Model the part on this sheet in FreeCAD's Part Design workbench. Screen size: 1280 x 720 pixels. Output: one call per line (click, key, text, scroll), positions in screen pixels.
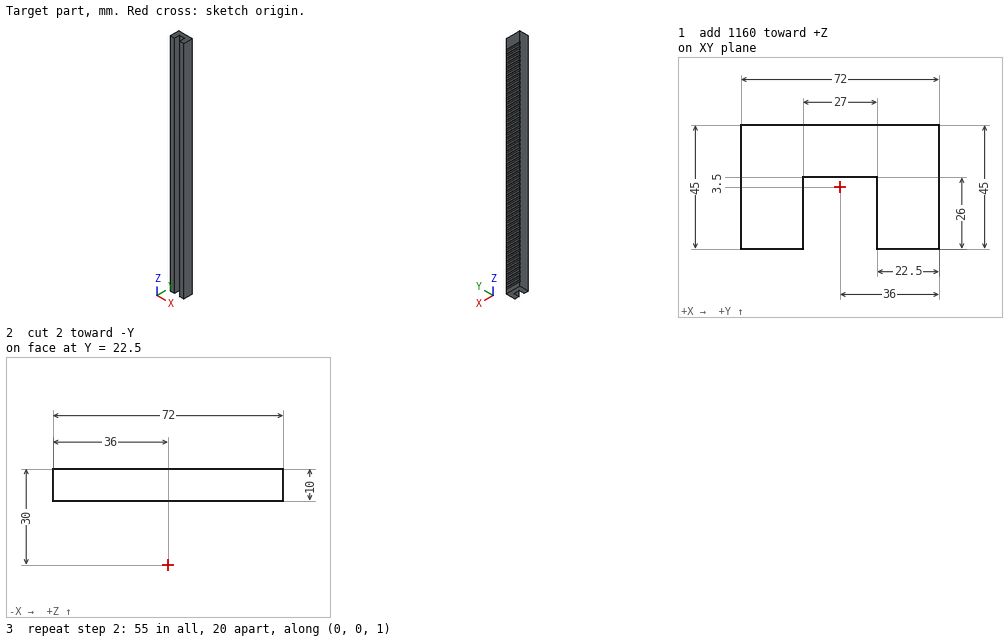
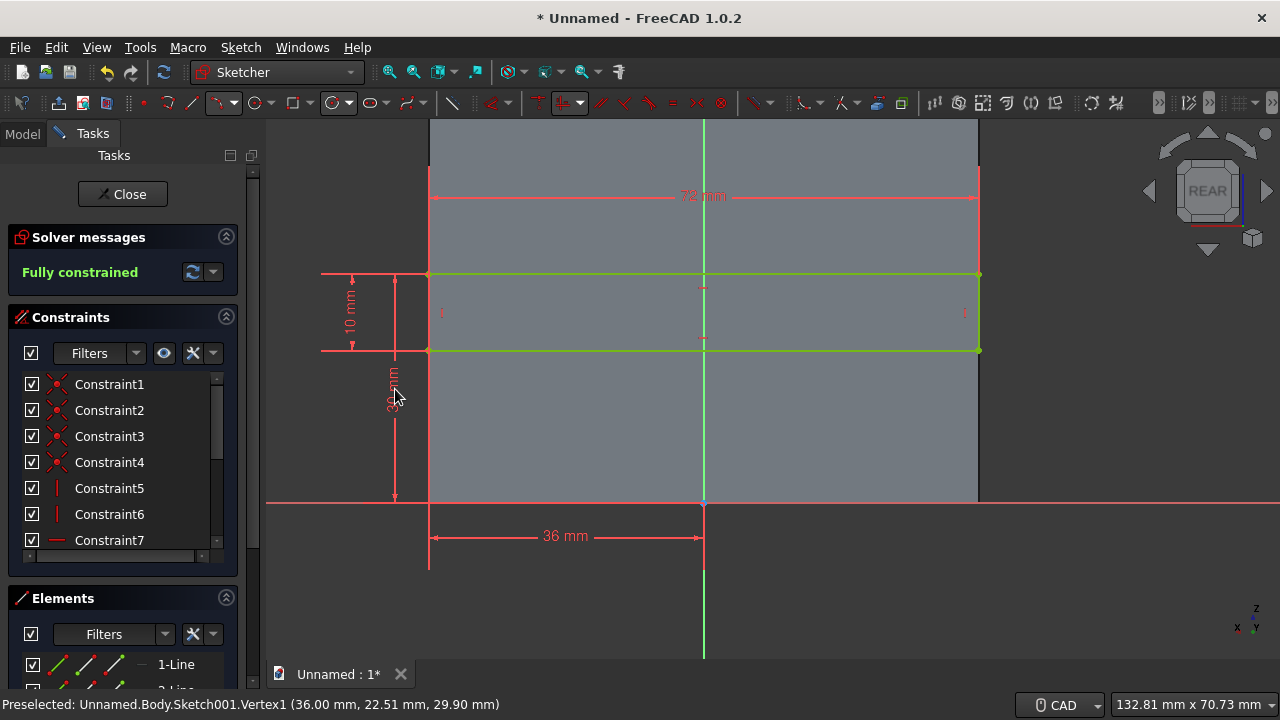
click(123, 194)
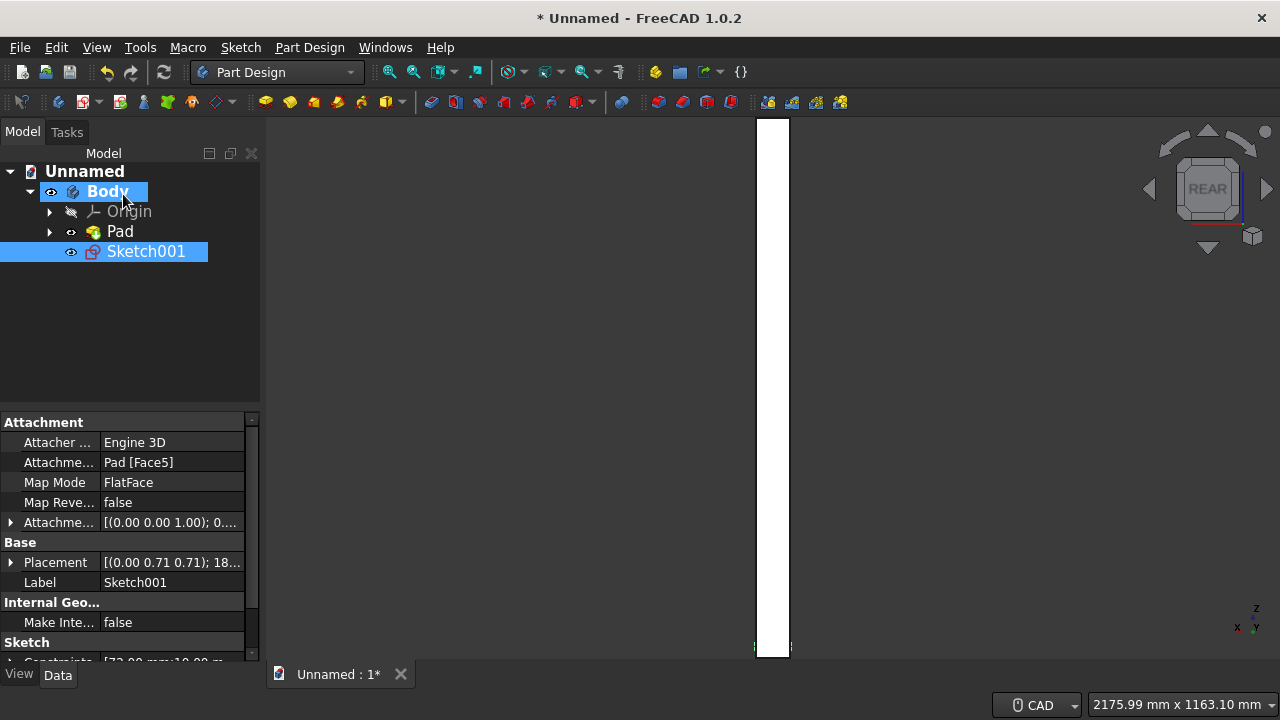
click(432, 102)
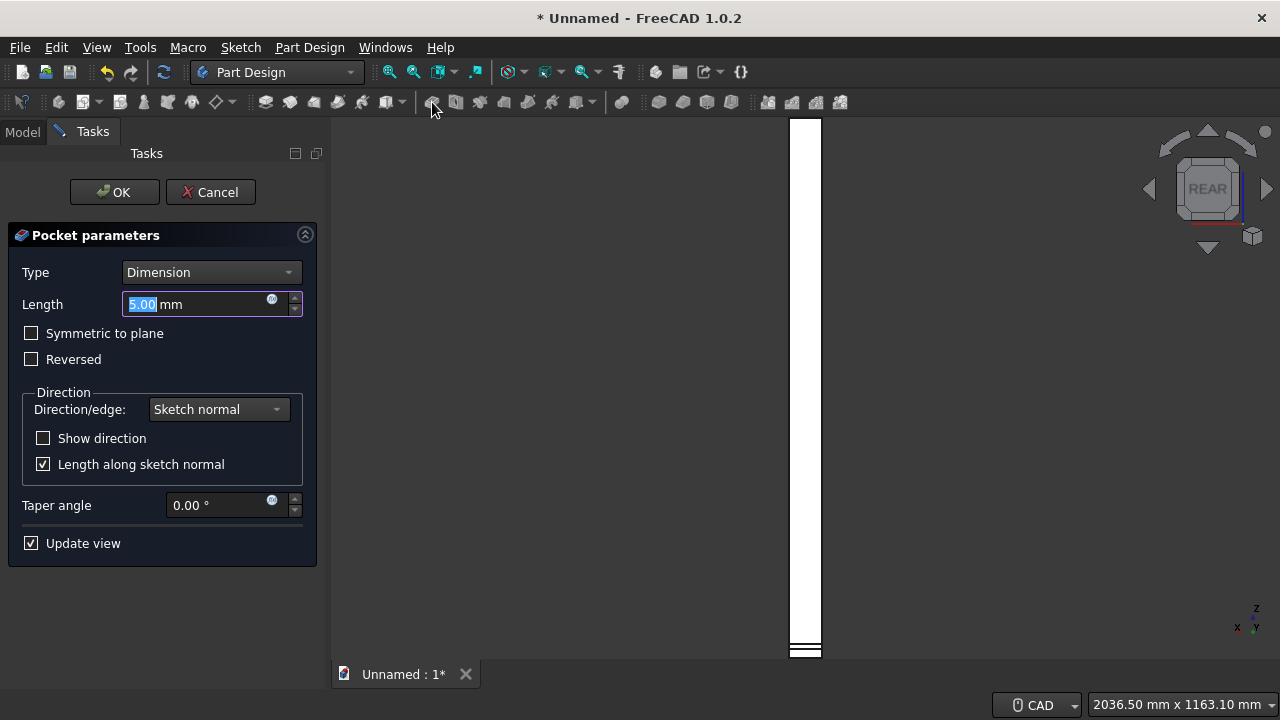
text(2)
key(Tab)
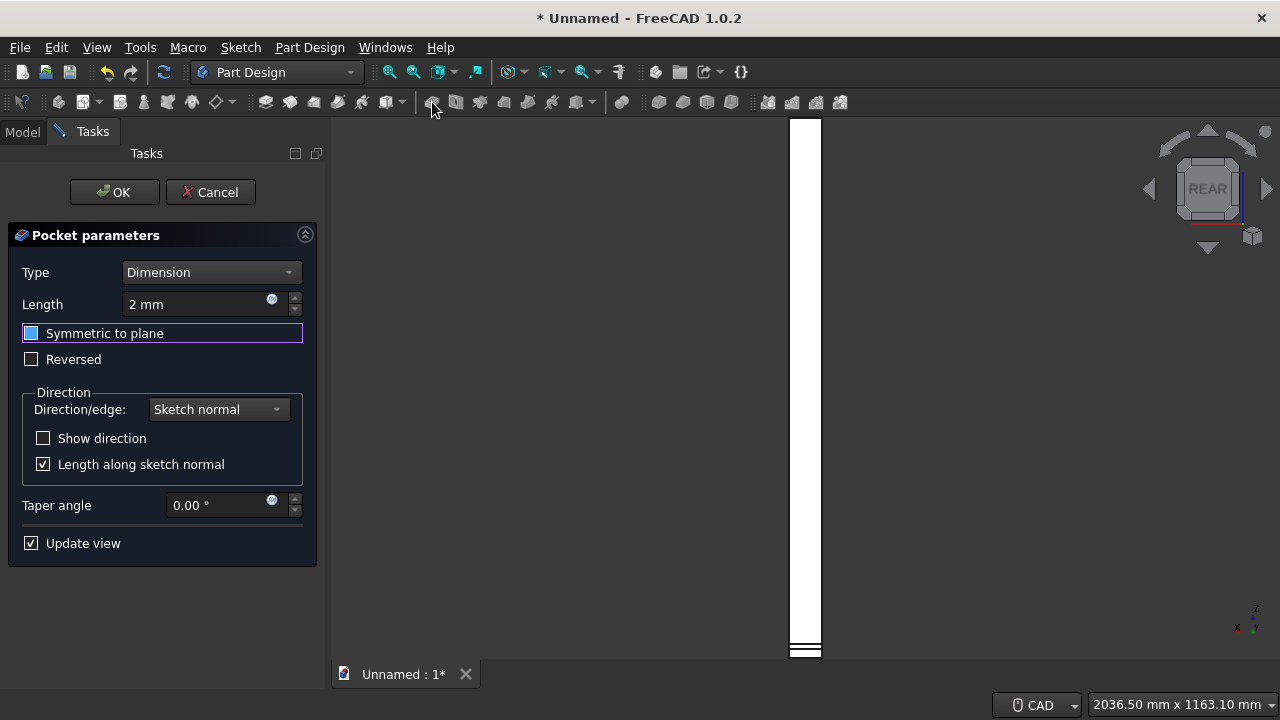
click(115, 192)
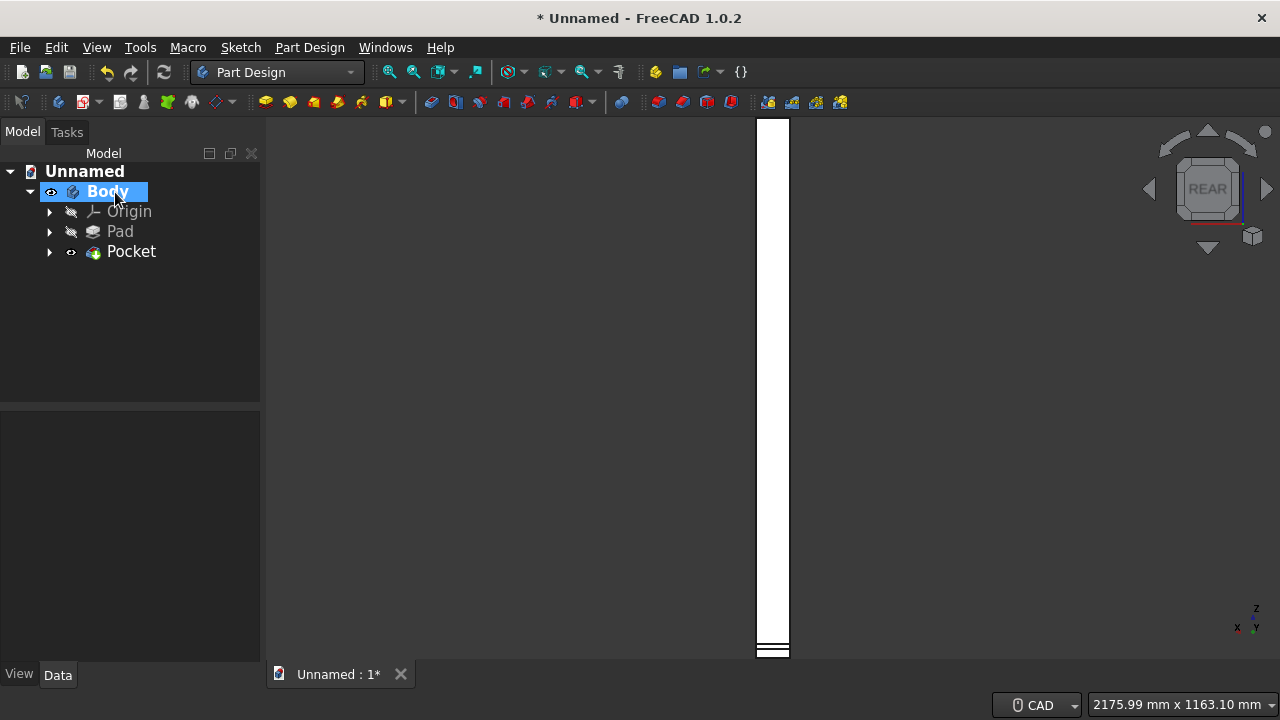
click(116, 252)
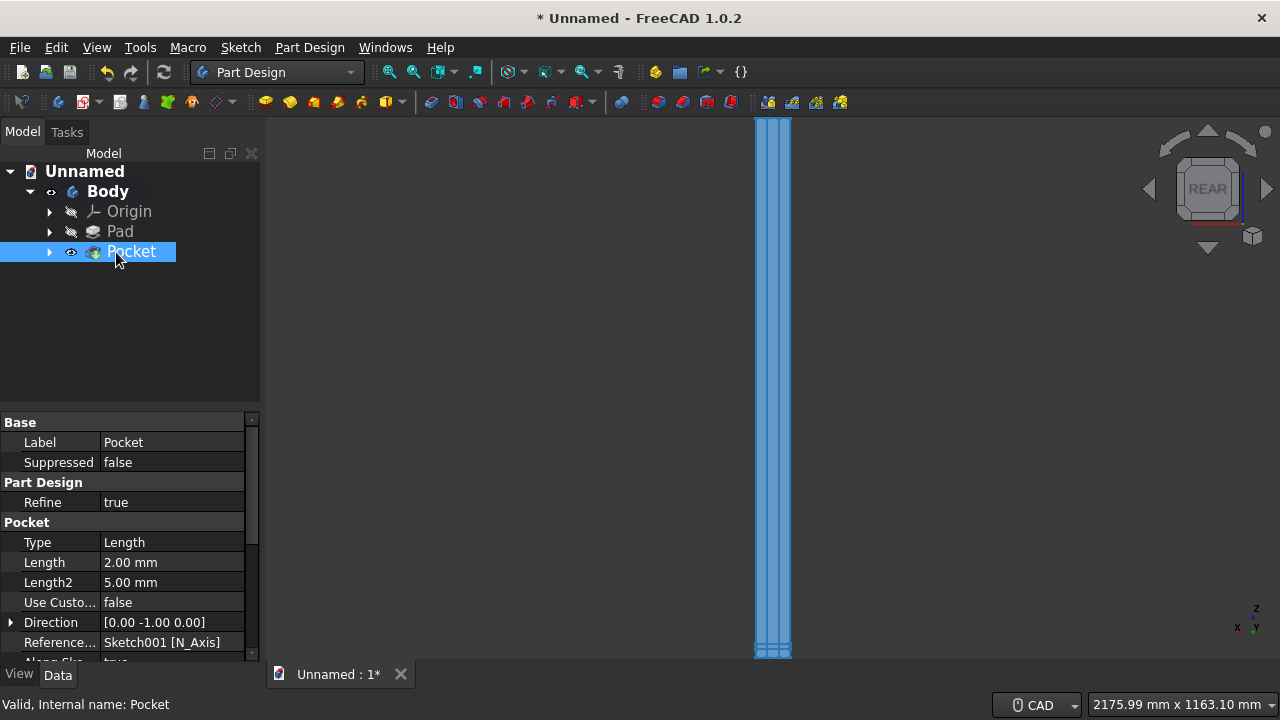
click(792, 102)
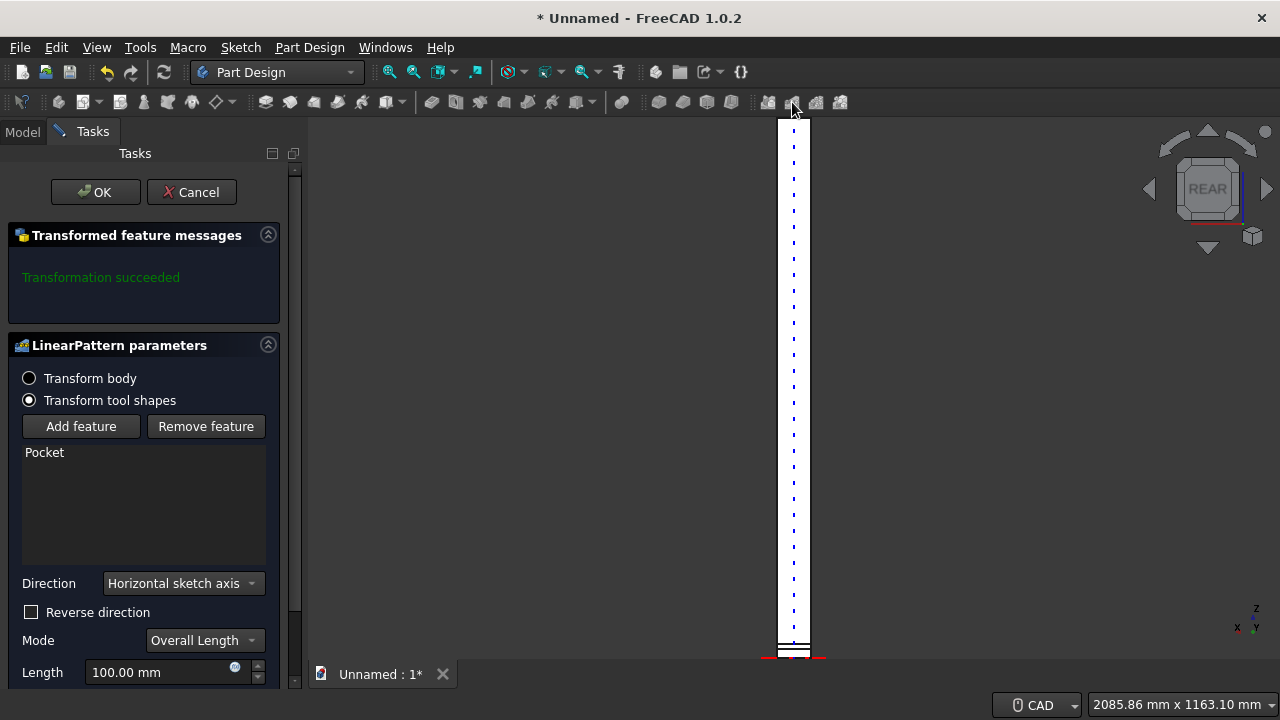
click(184, 584)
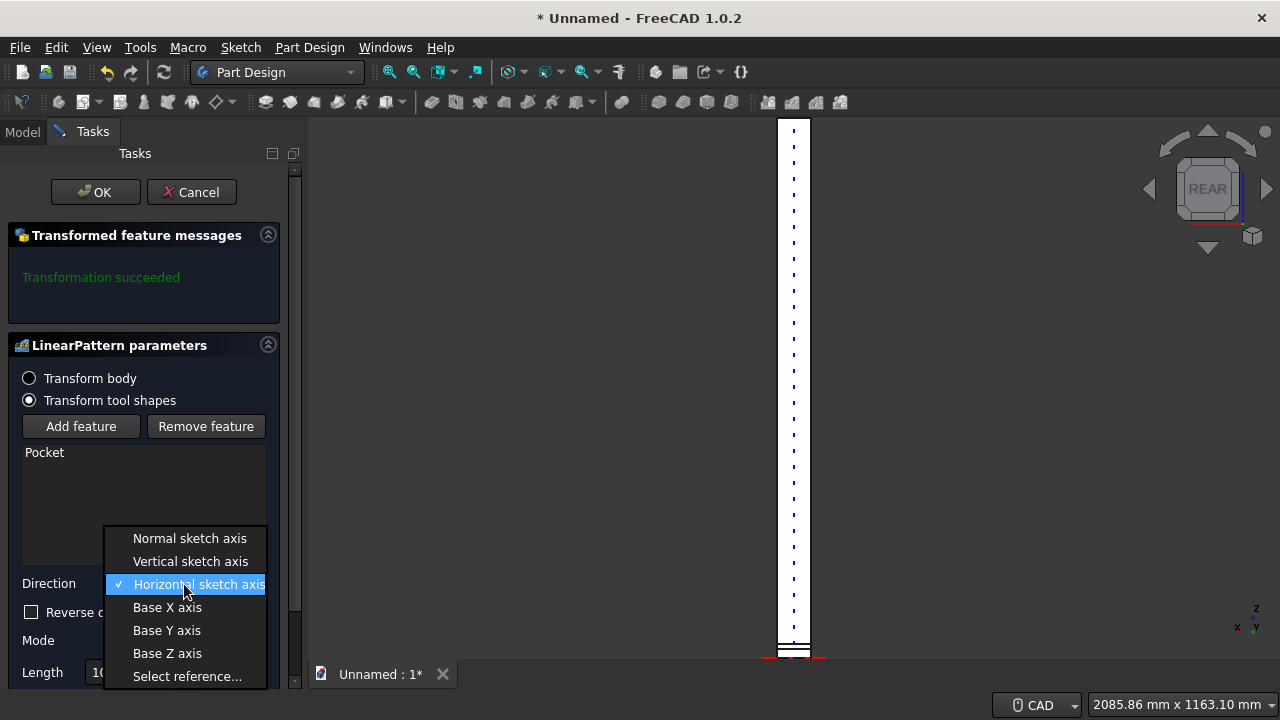
click(184, 654)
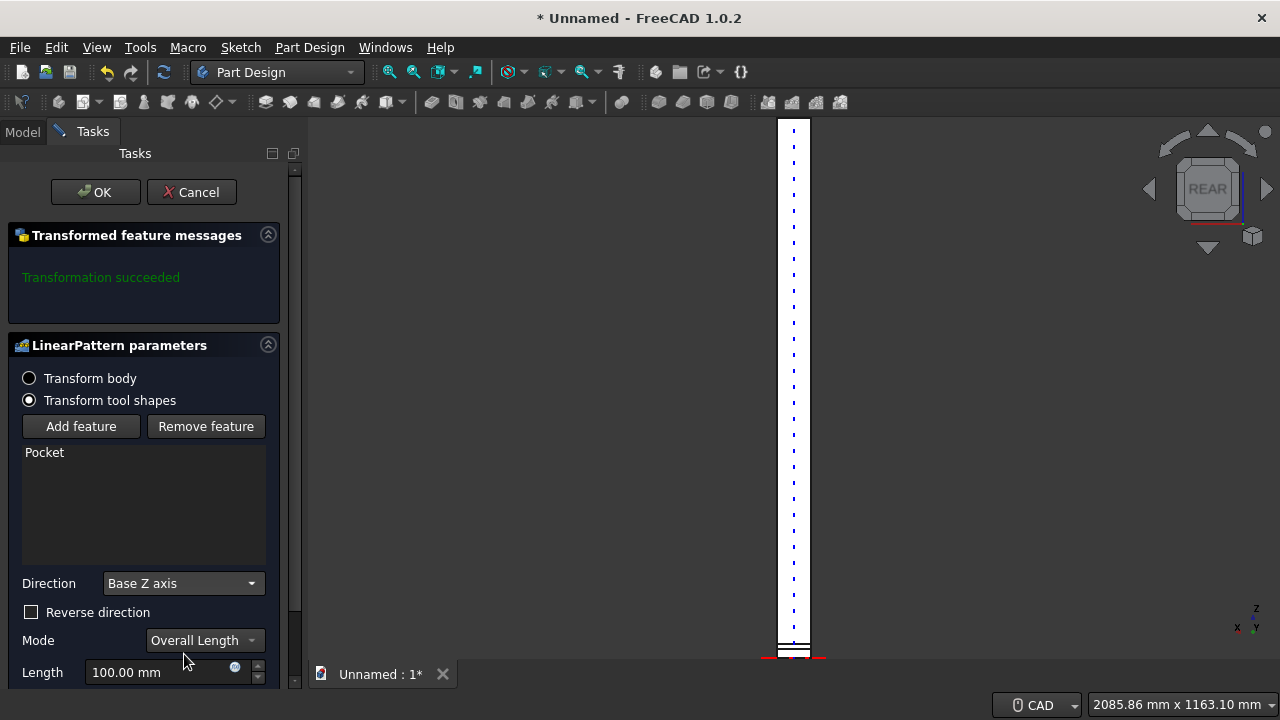
click(206, 640)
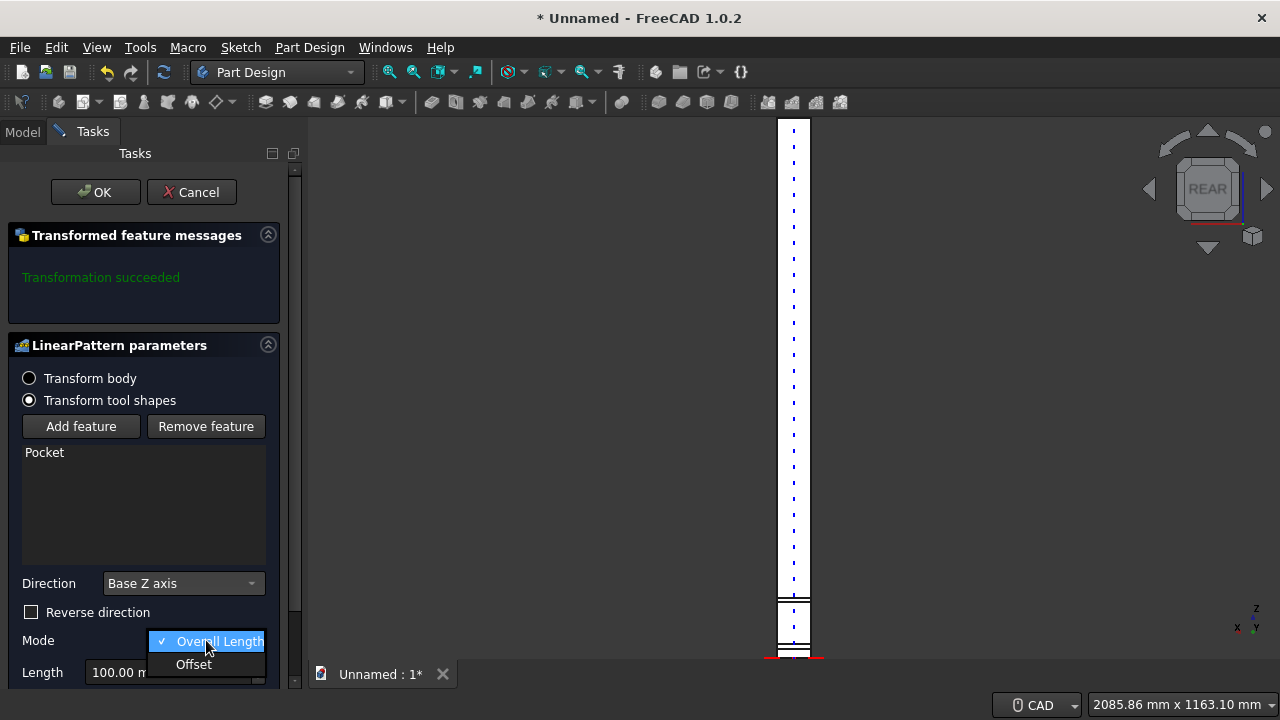
click(206, 664)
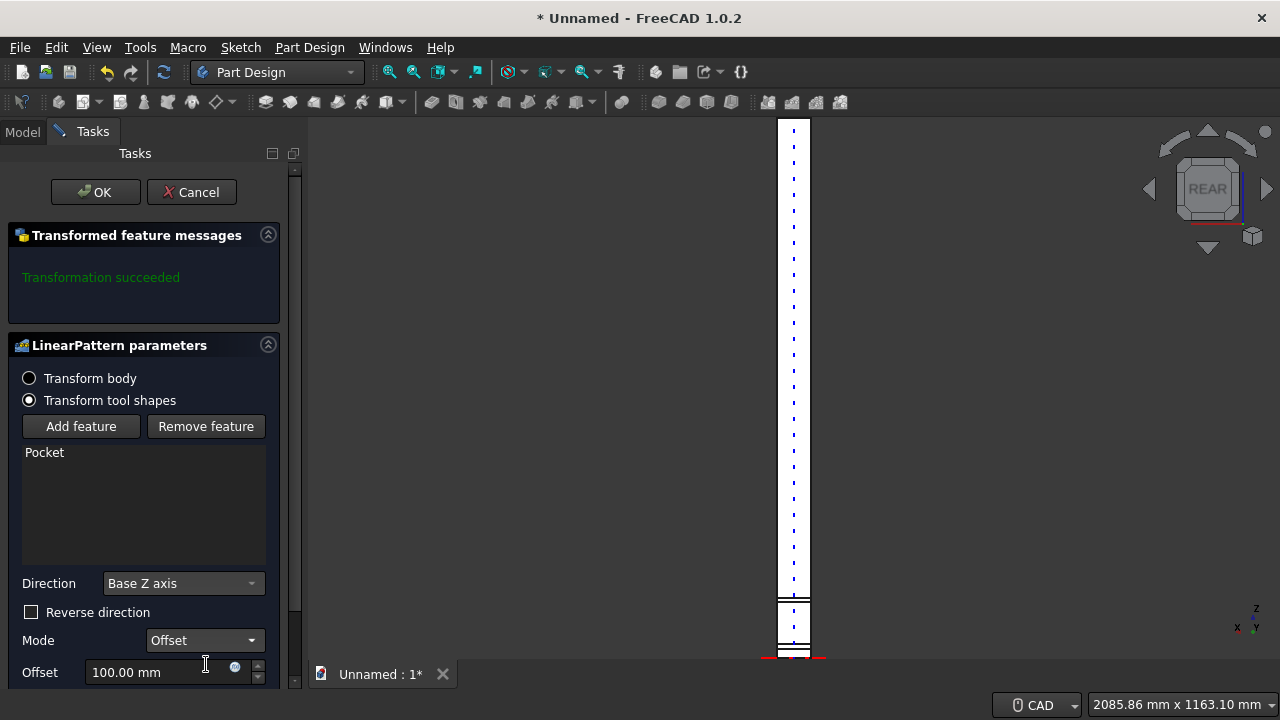
triple_click(168, 672)